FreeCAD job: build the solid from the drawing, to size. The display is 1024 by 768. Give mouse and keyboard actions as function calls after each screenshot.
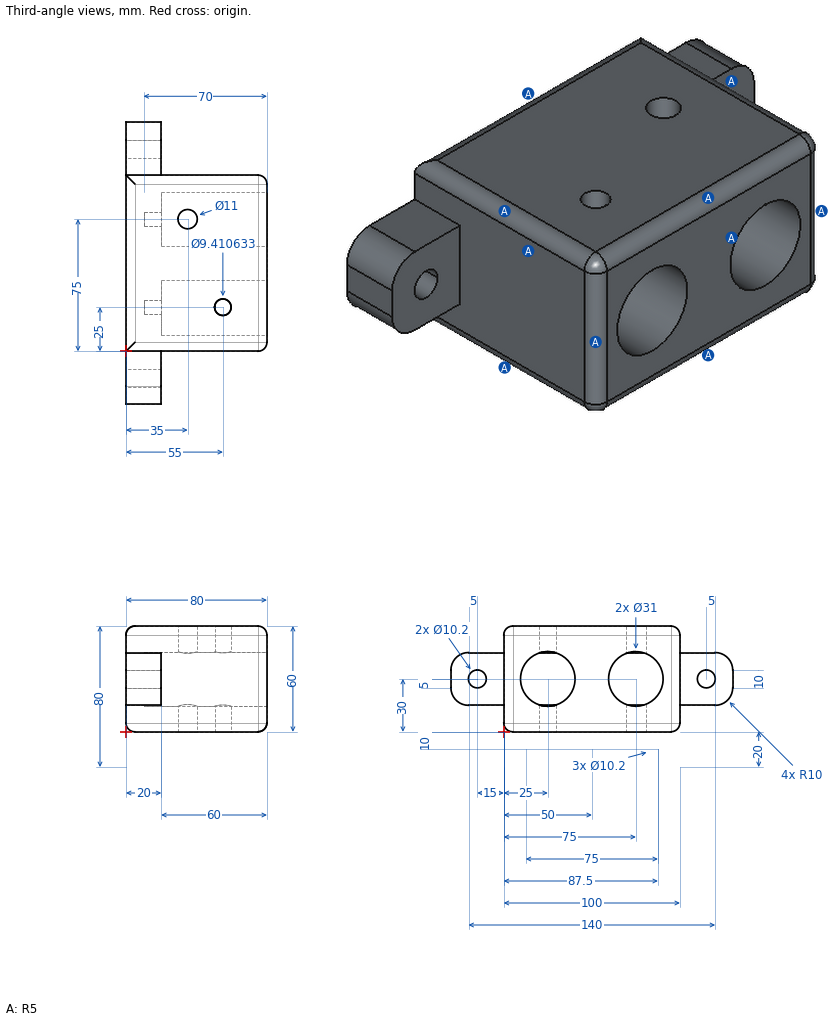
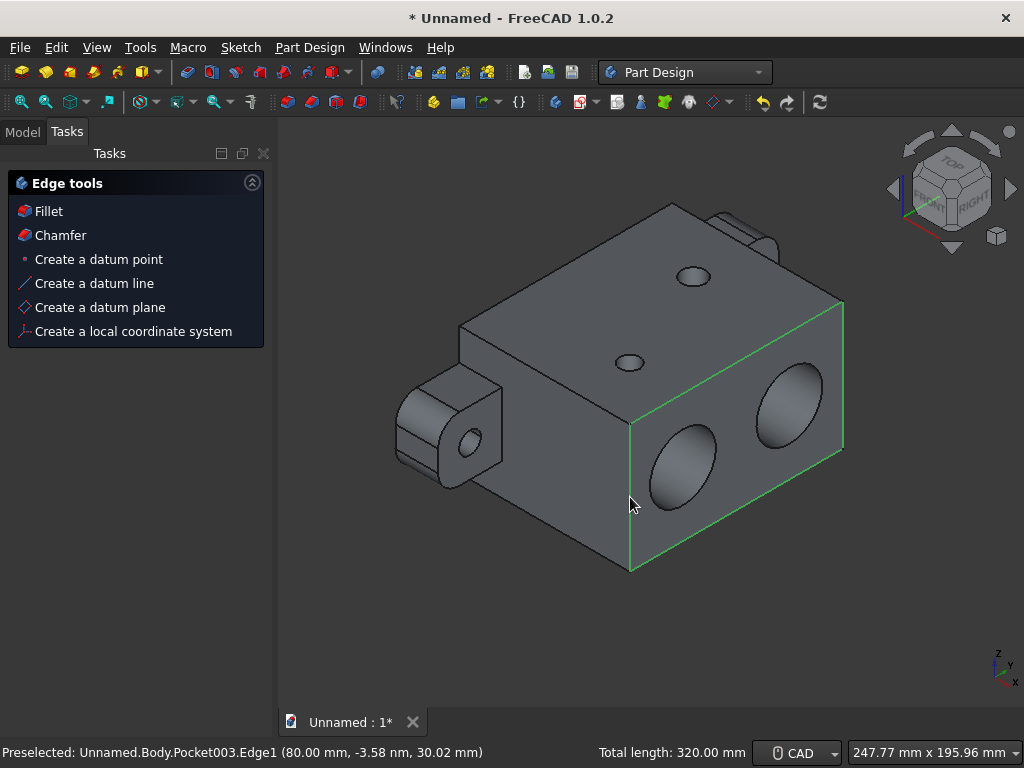
click(545, 374, ctrl)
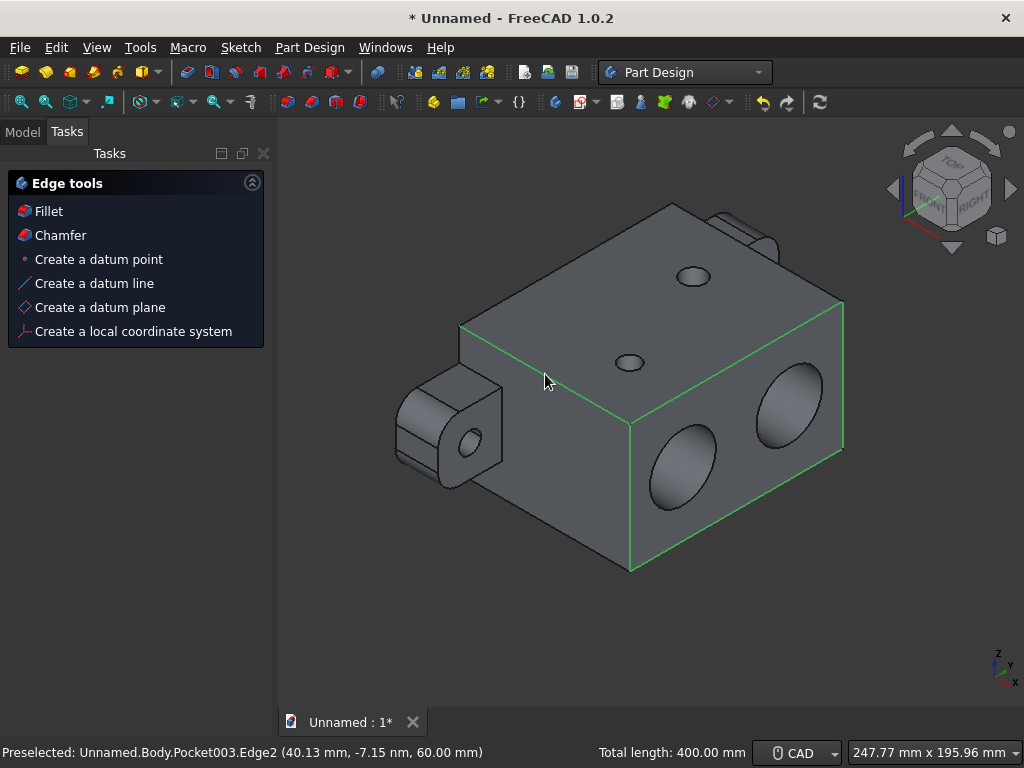
key(2)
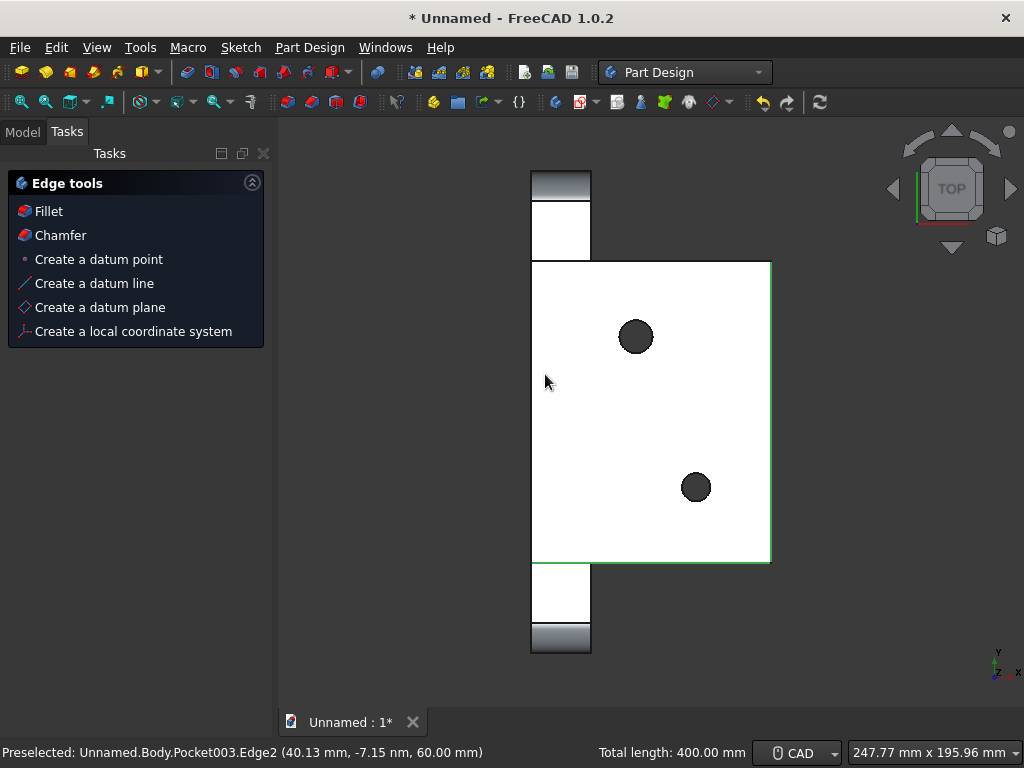
click(531, 411, ctrl)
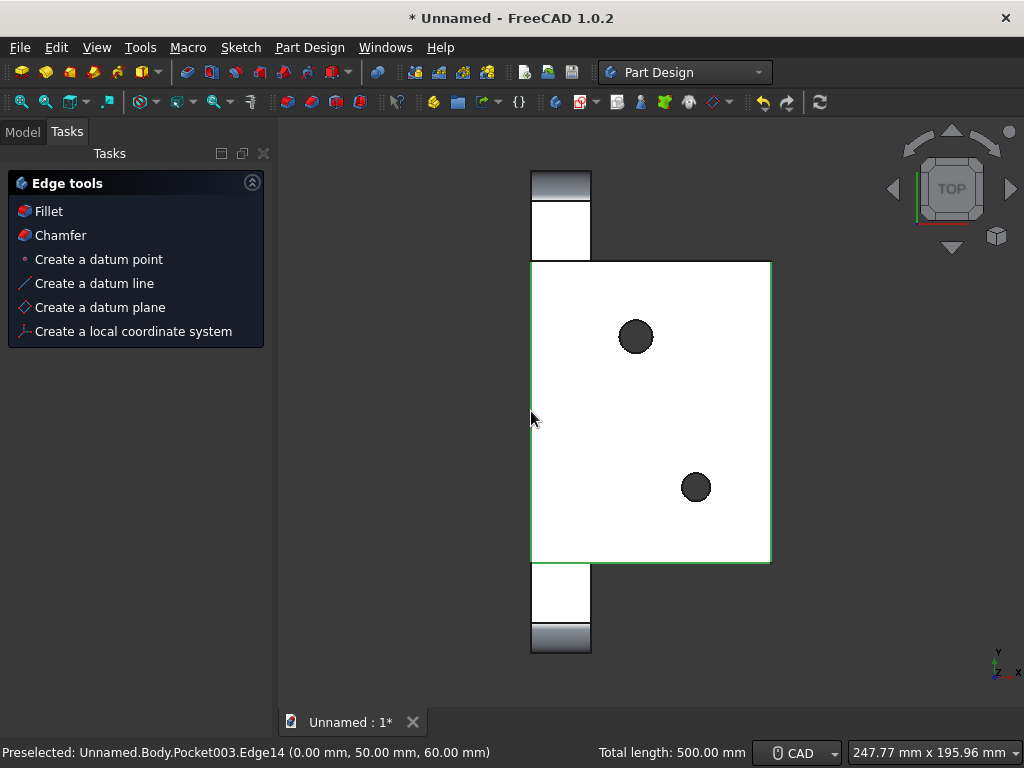
click(651, 260, ctrl)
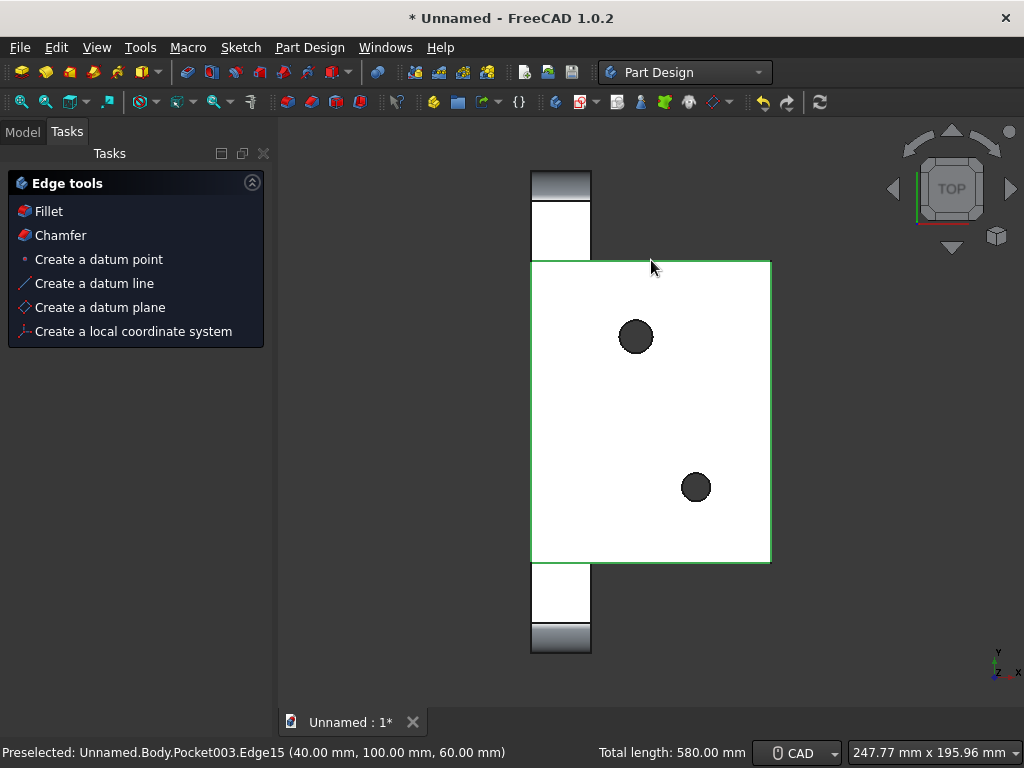
key(1)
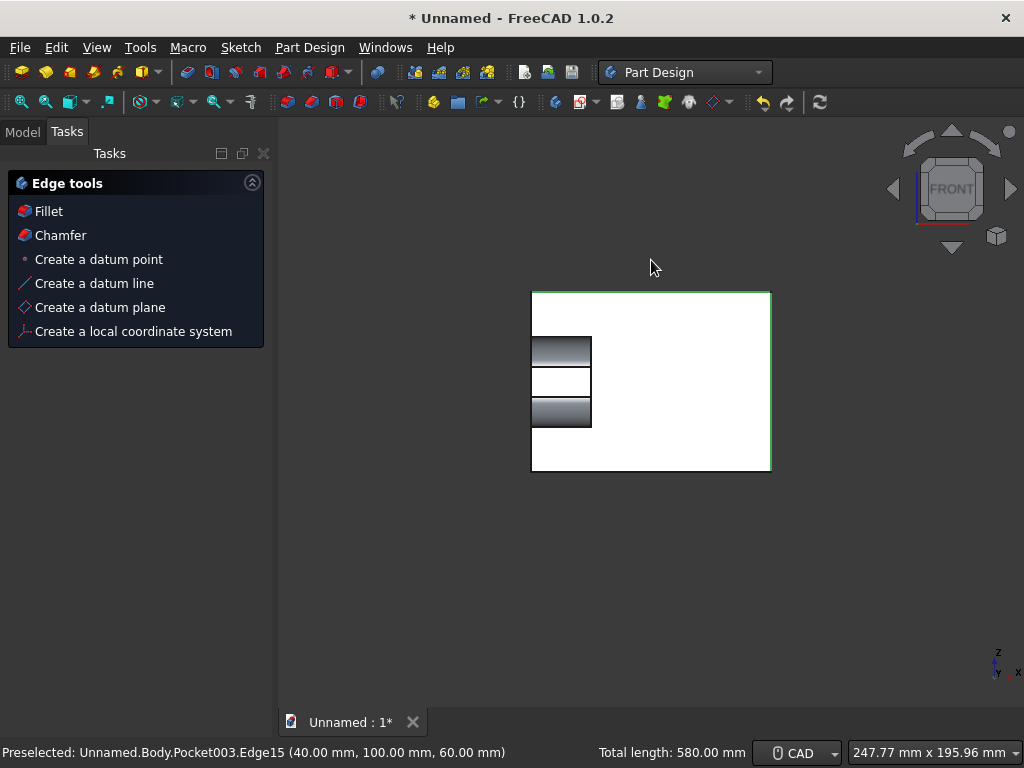
key(v)
key(f)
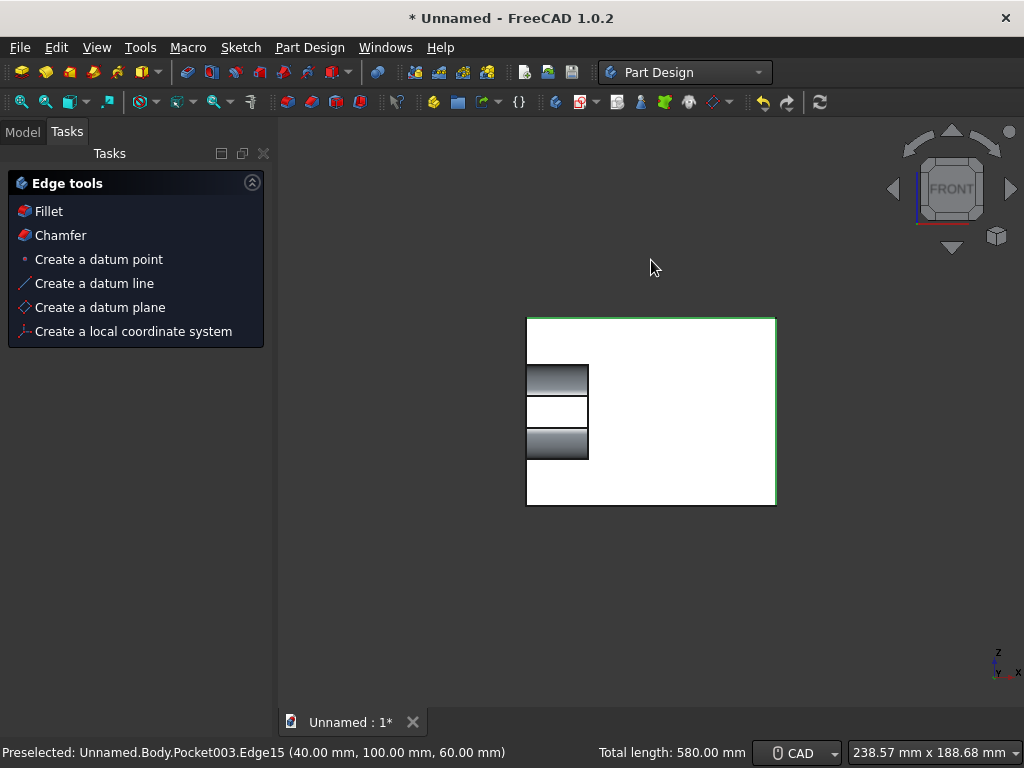
key(3)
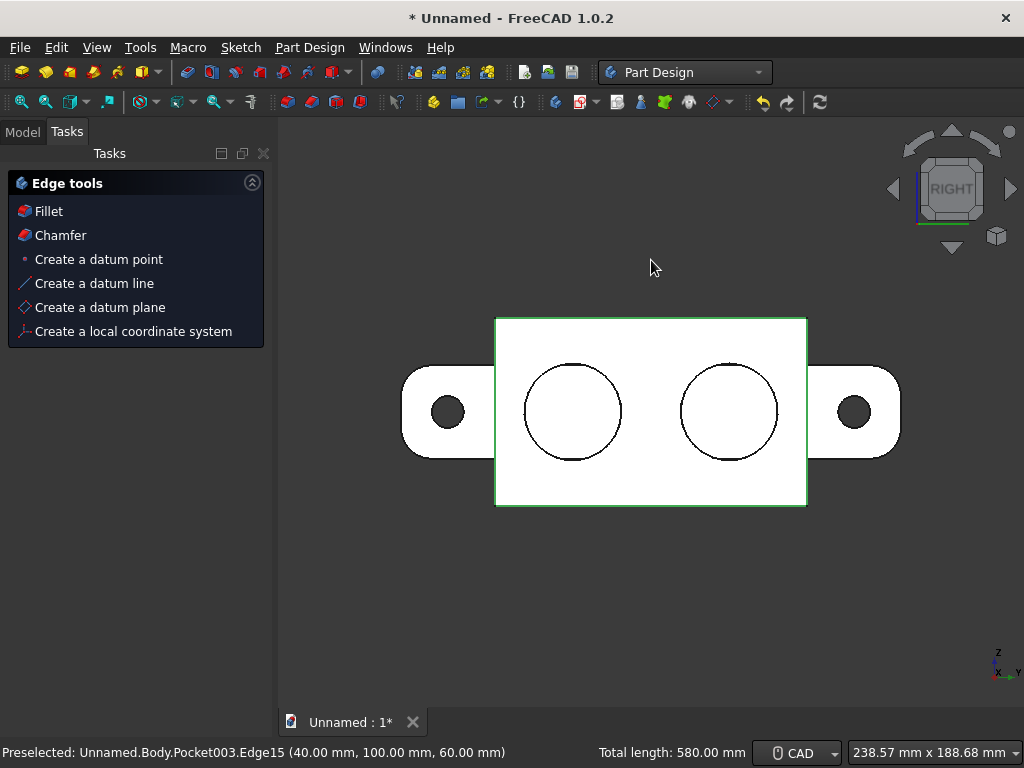
key(5)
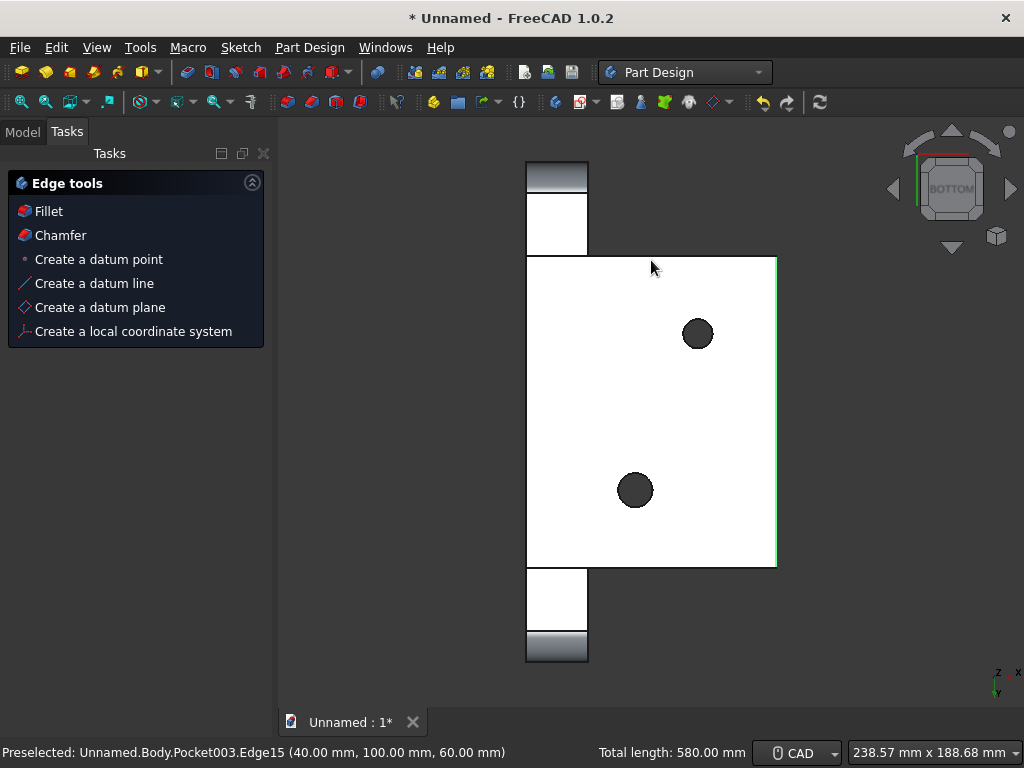
click(651, 255, ctrl)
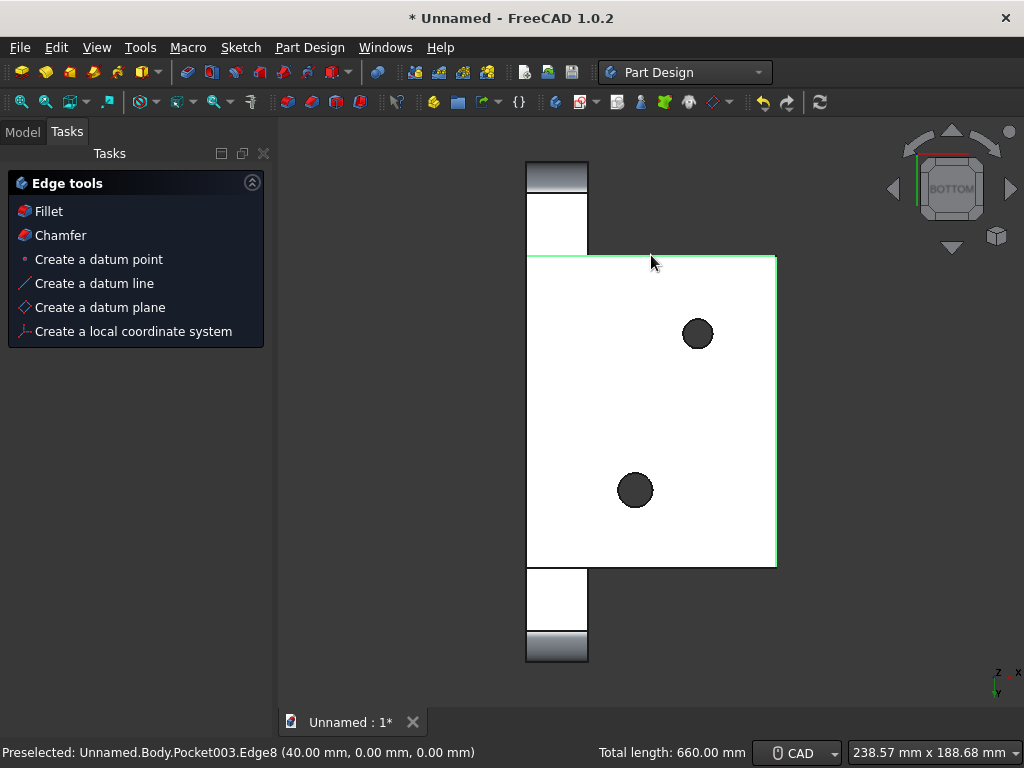
key(4)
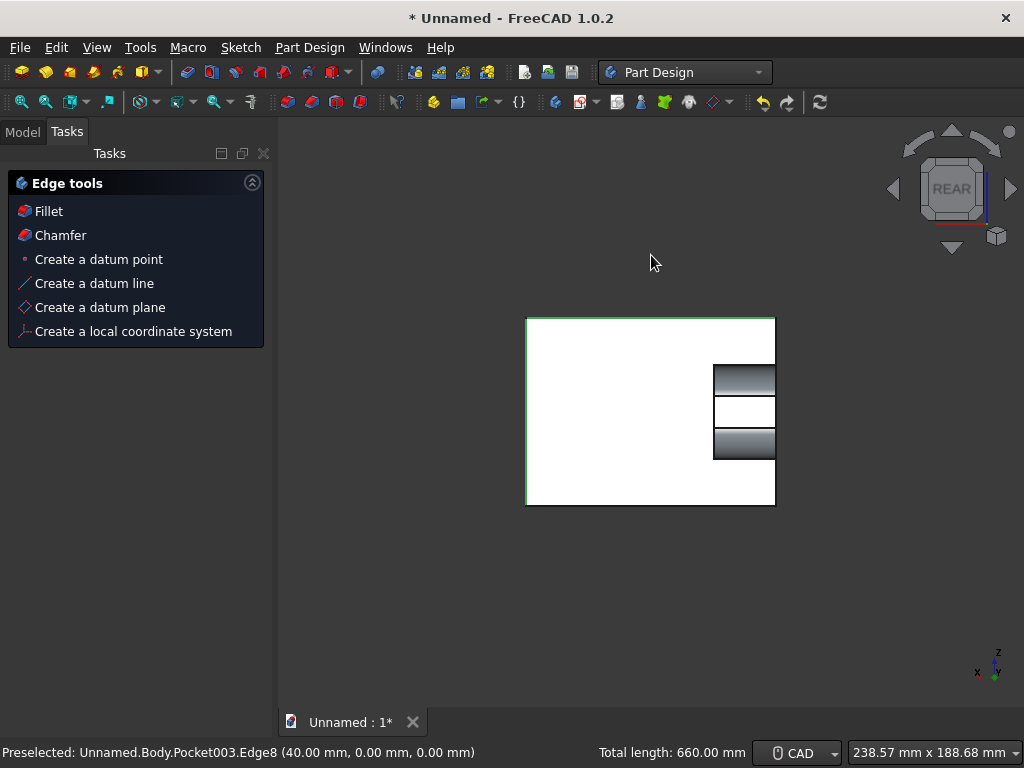
key(v)
key(f)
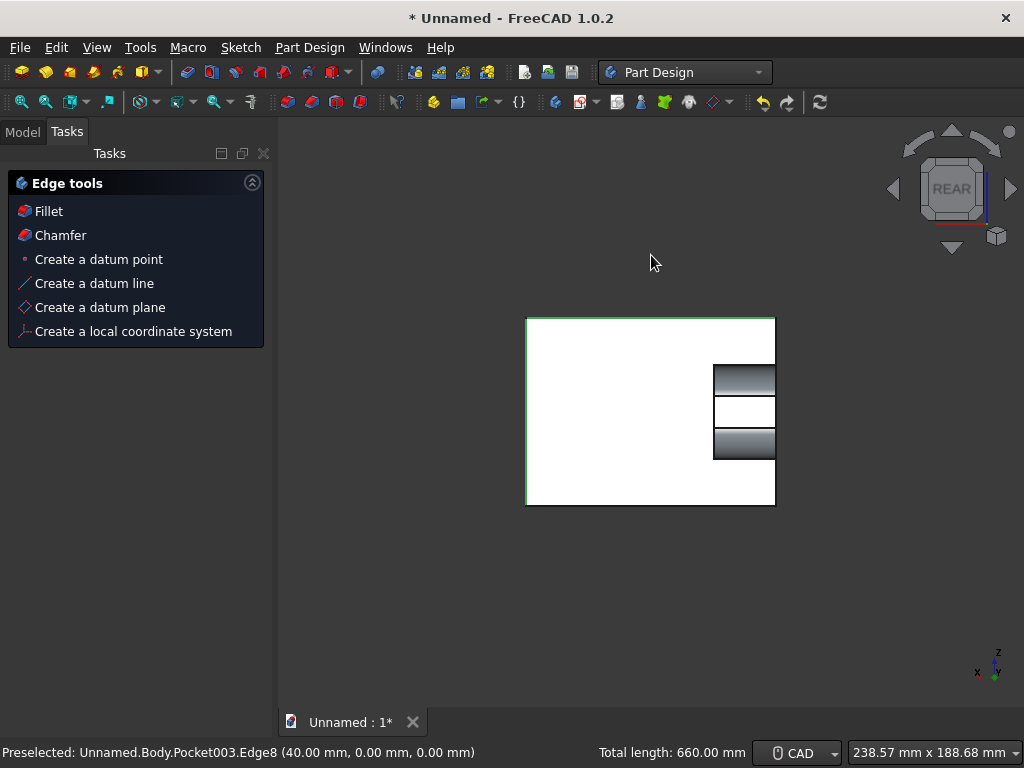
click(651, 505, ctrl)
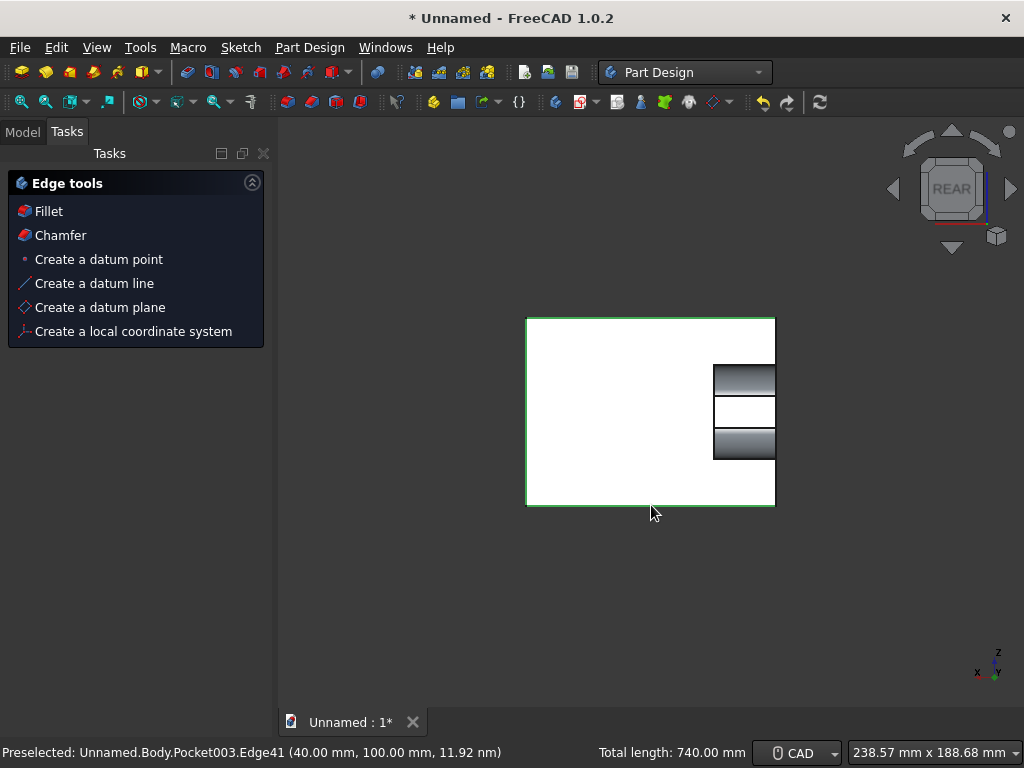
key(6)